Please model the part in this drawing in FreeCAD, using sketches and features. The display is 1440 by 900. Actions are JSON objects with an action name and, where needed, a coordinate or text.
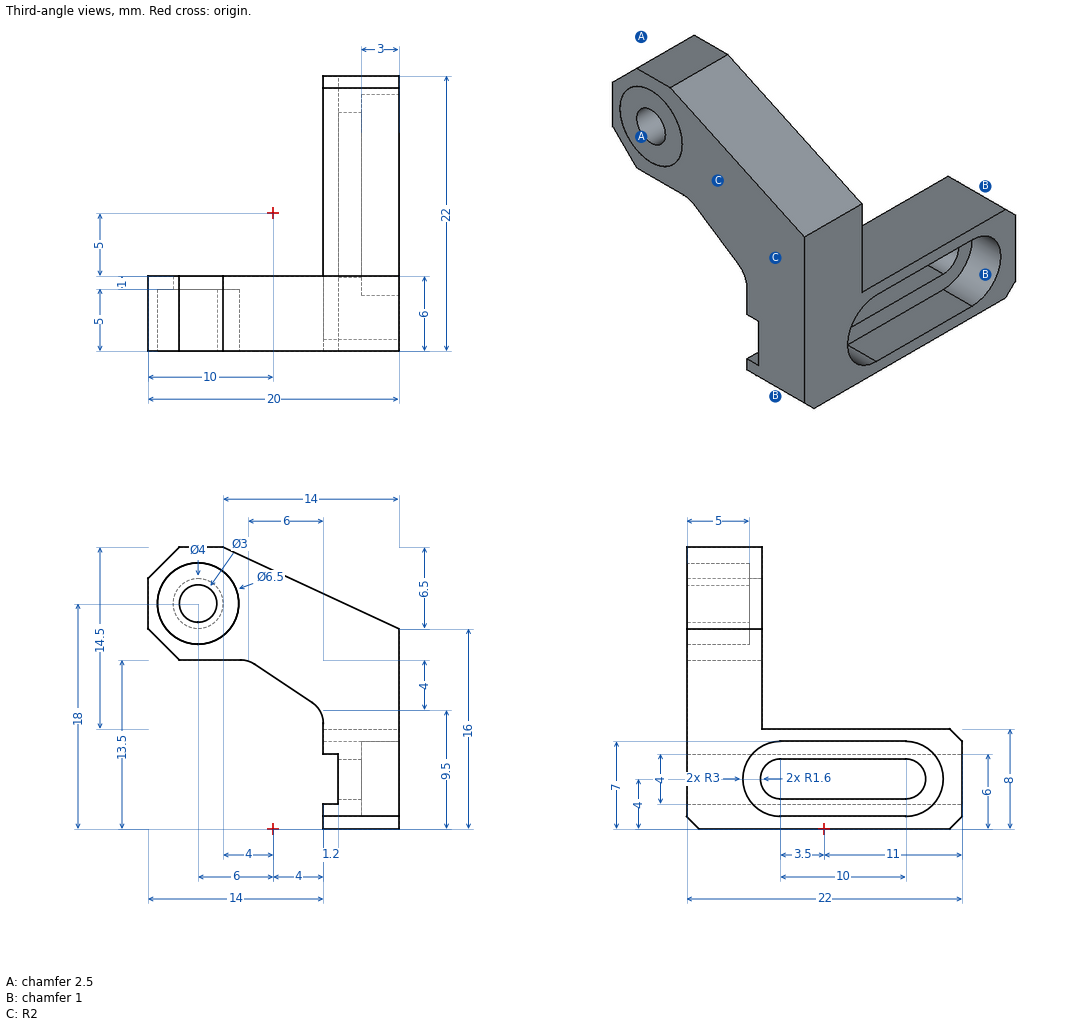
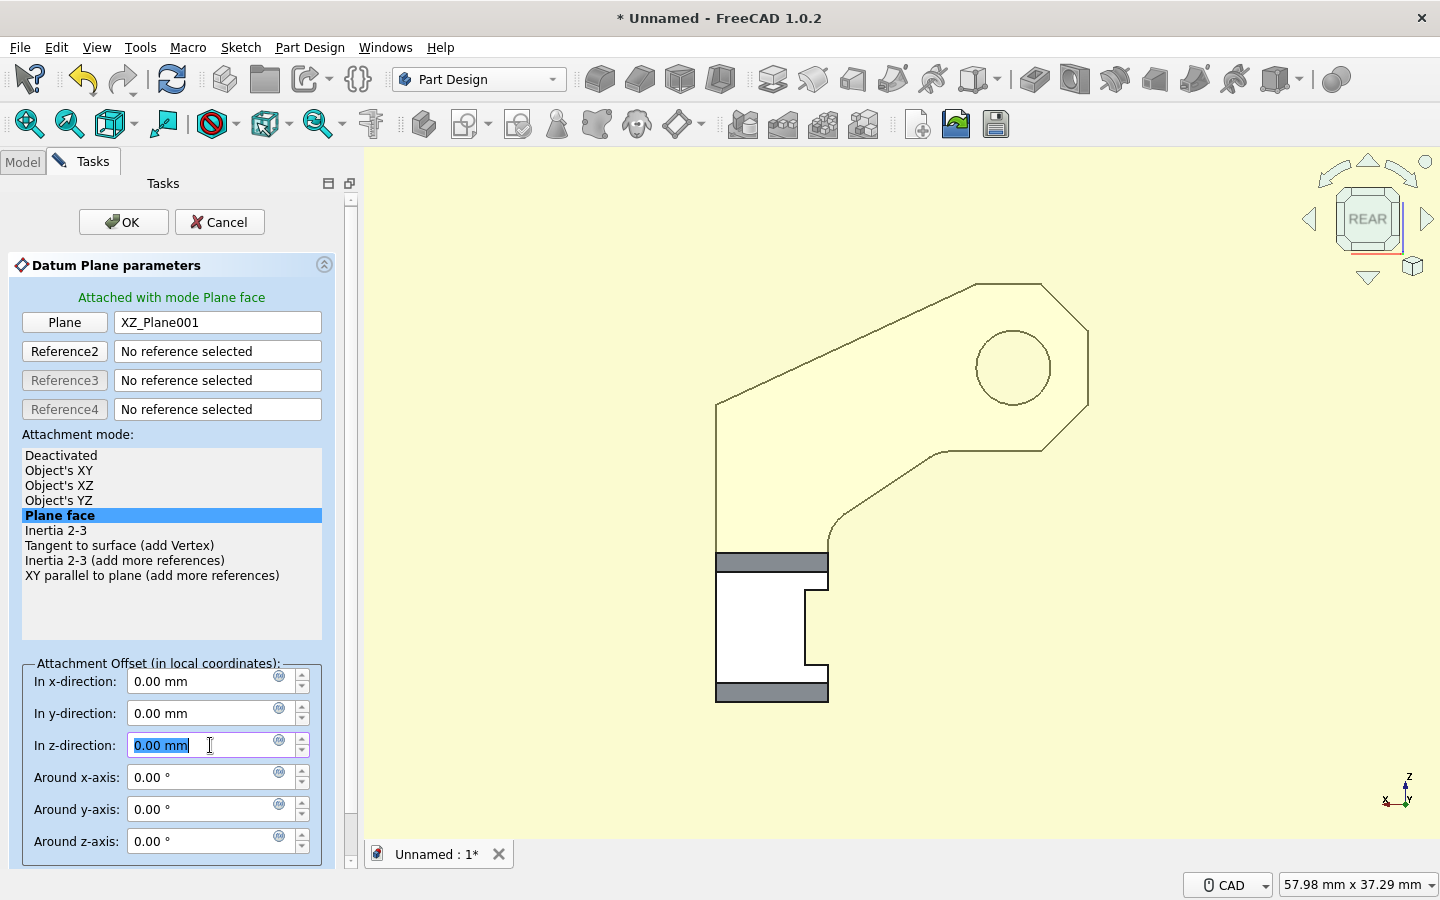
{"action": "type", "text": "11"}
{"action": "key", "text": "Tab"}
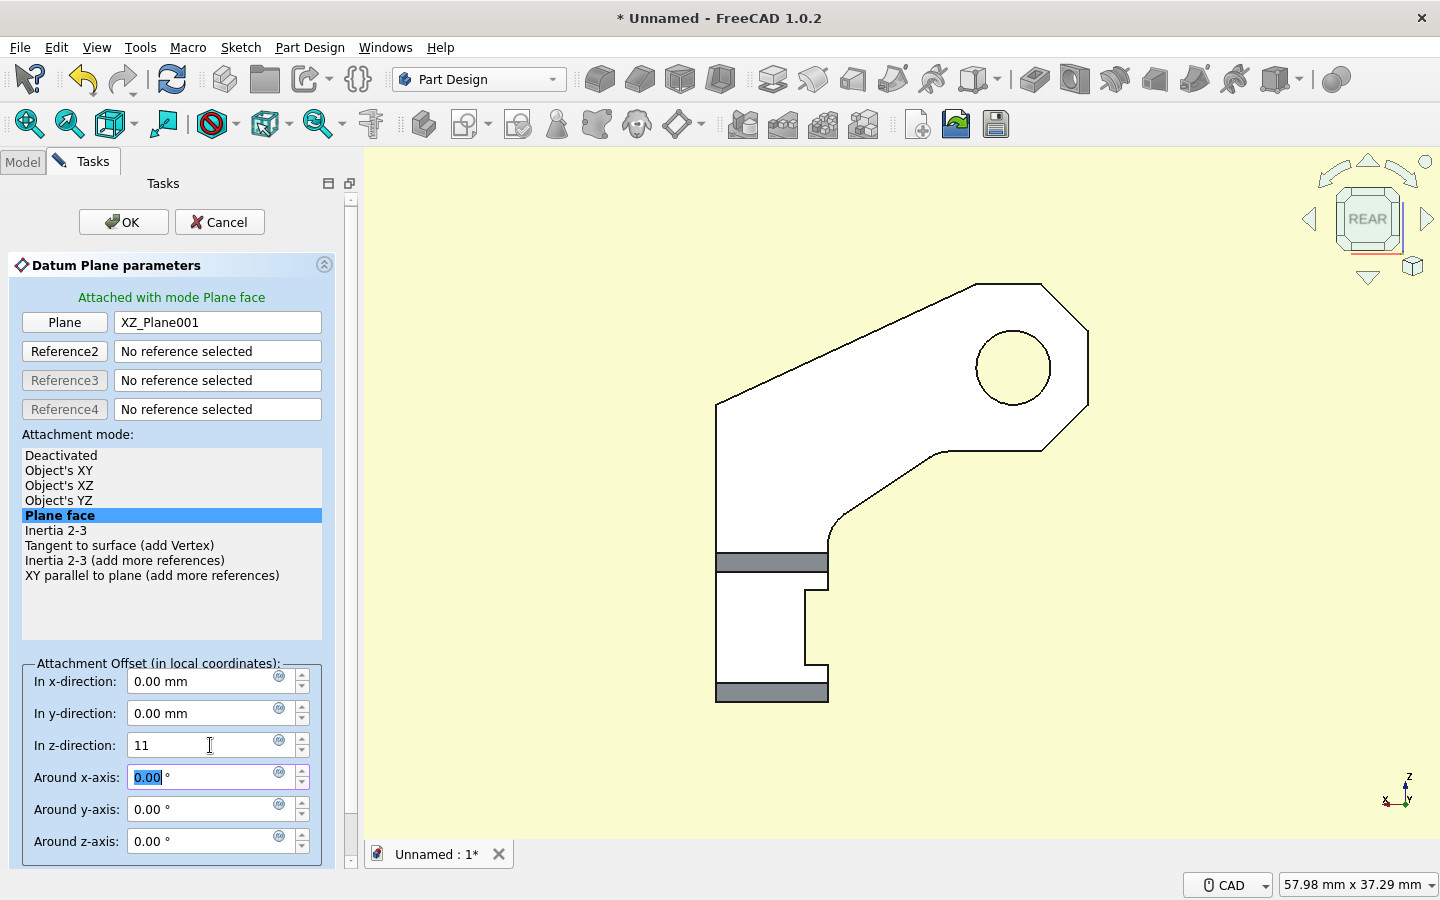
{"action": "left_click", "coordinate": [124, 222]}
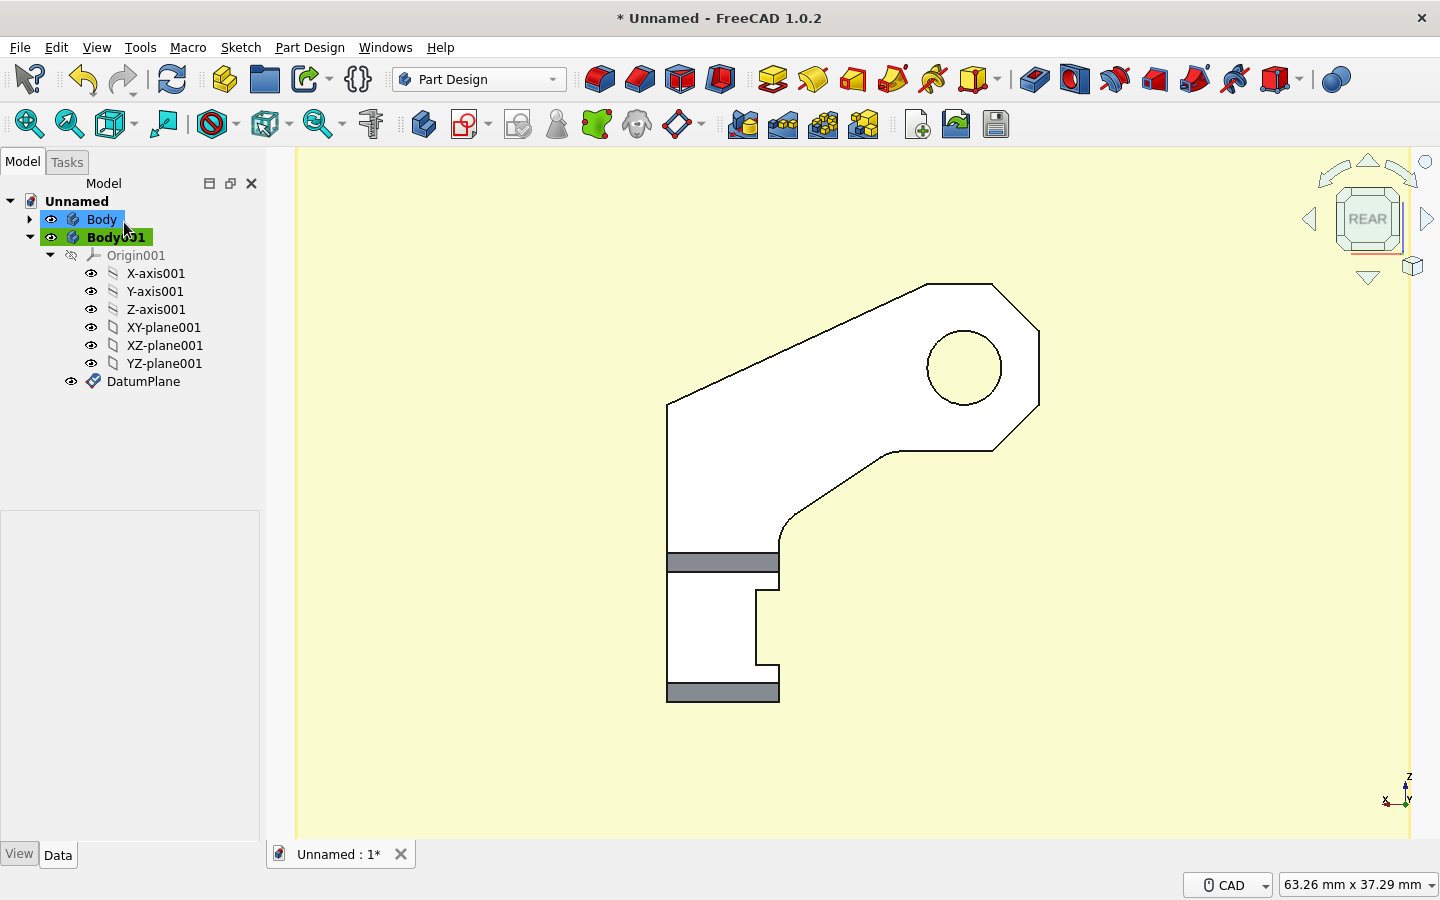
{"action": "left_click", "coordinate": [116, 381]}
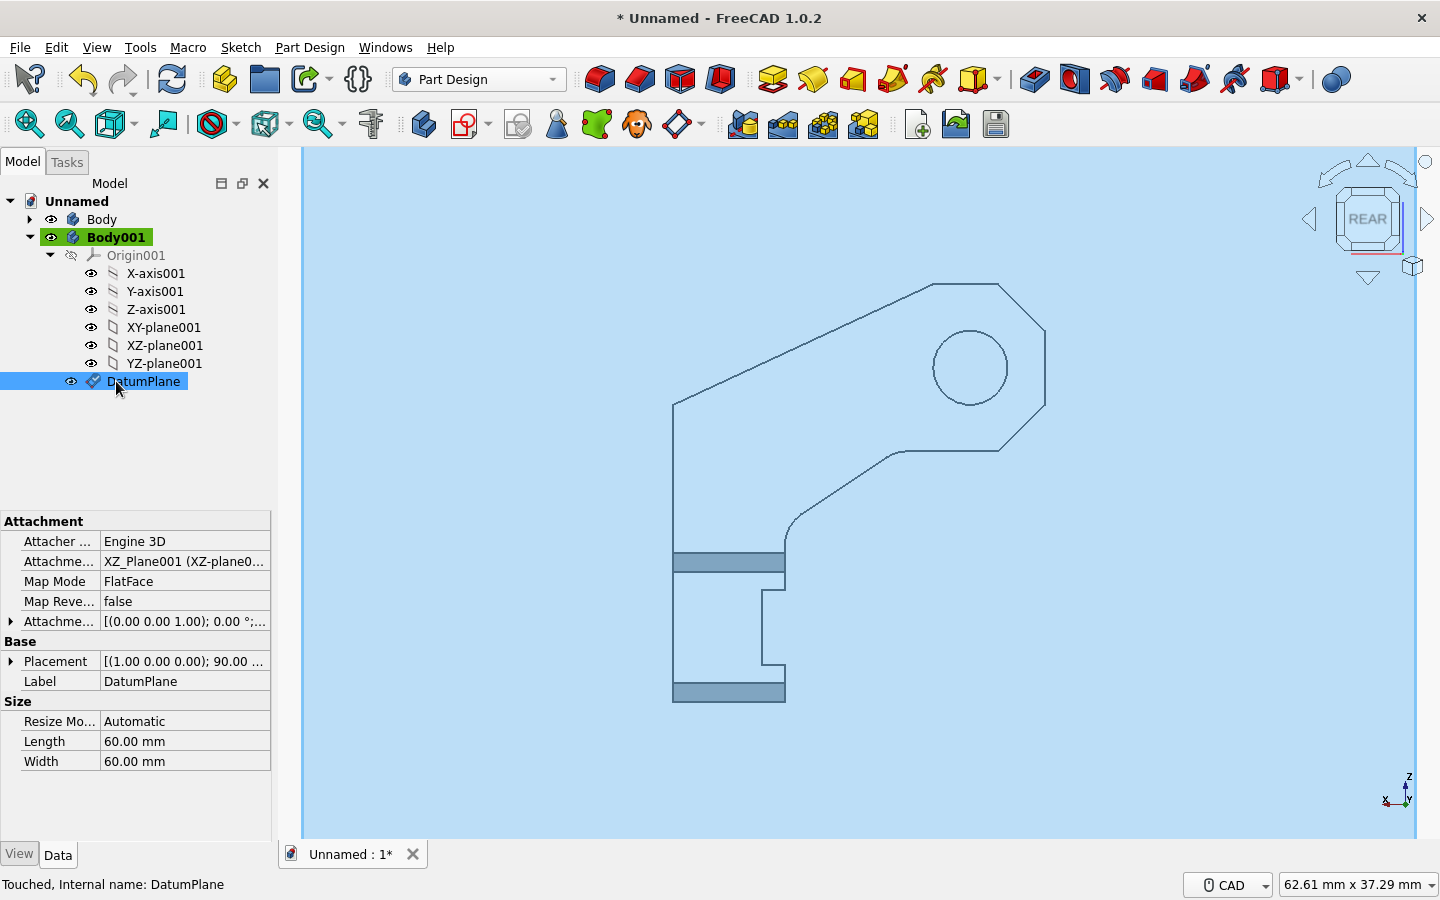
{"action": "left_click", "coordinate": [464, 124]}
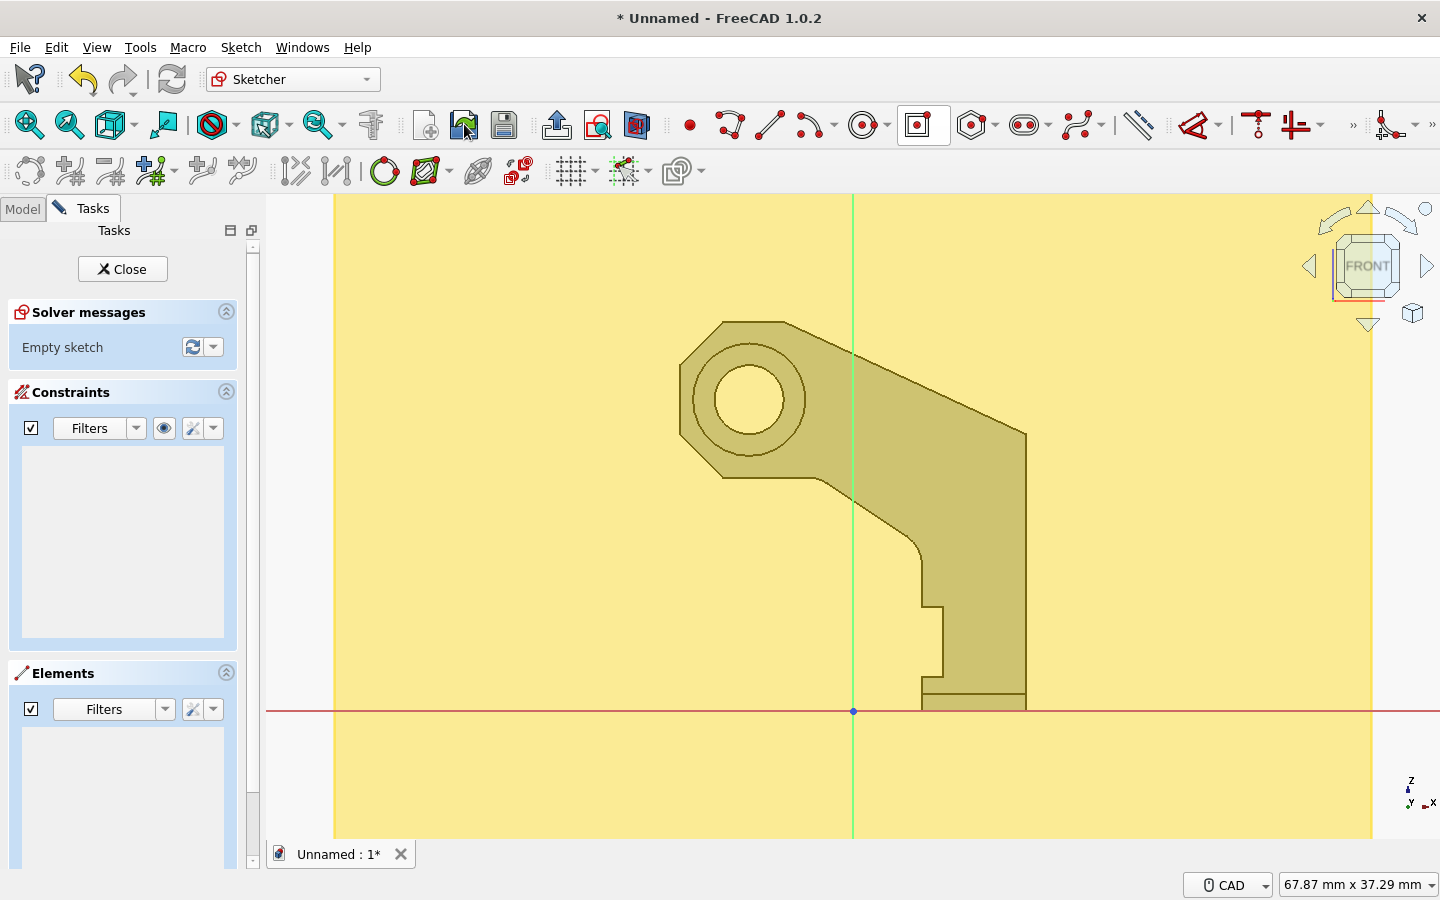
{"action": "scroll", "coordinate": [738, 362], "scroll_direction": "up", "scroll_amount": 7}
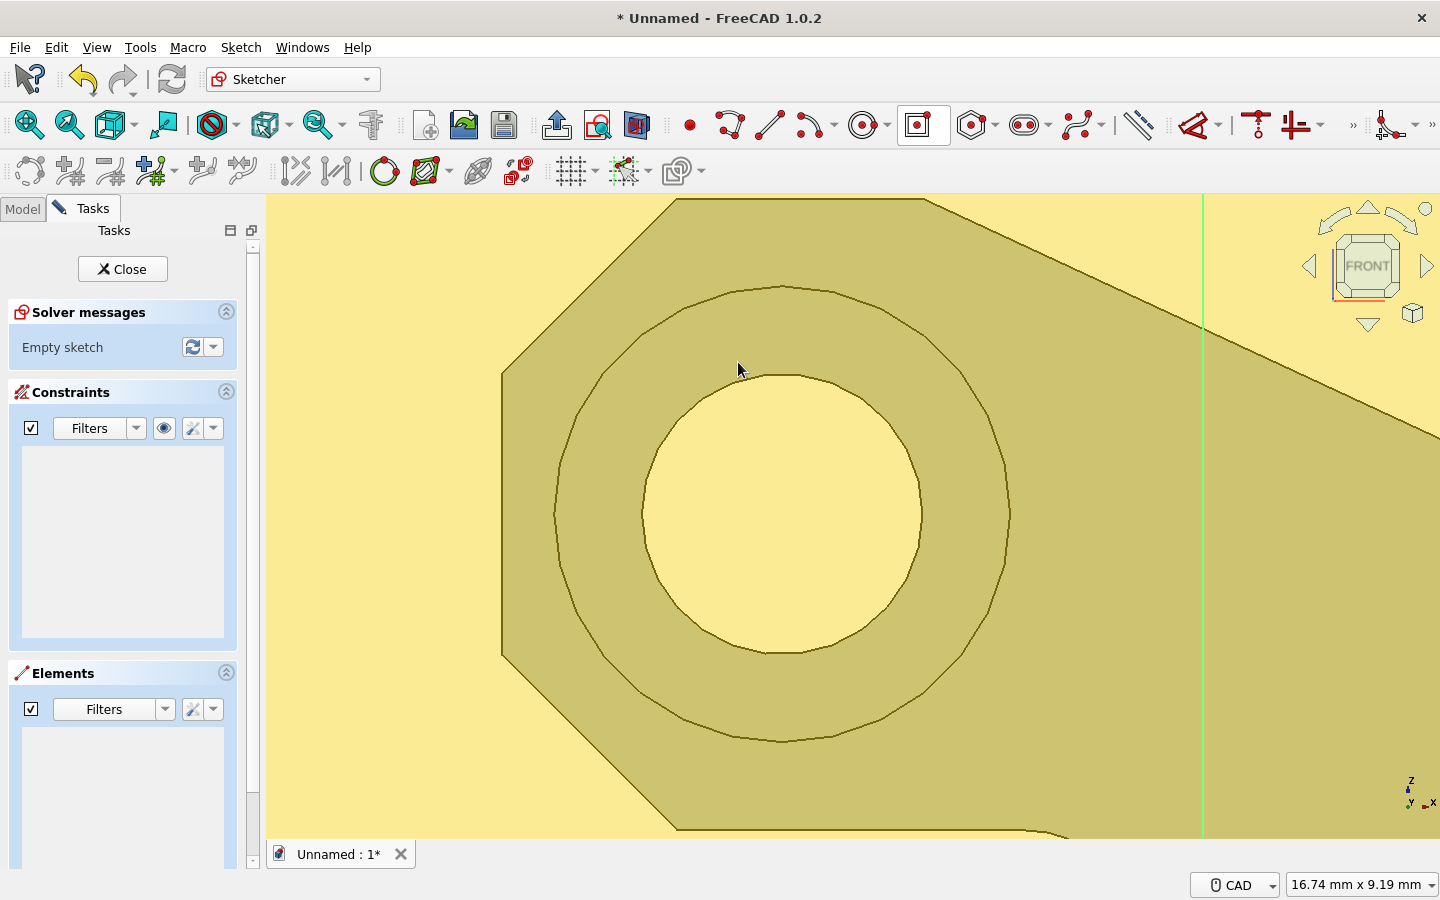
{"action": "left_click", "coordinate": [864, 126]}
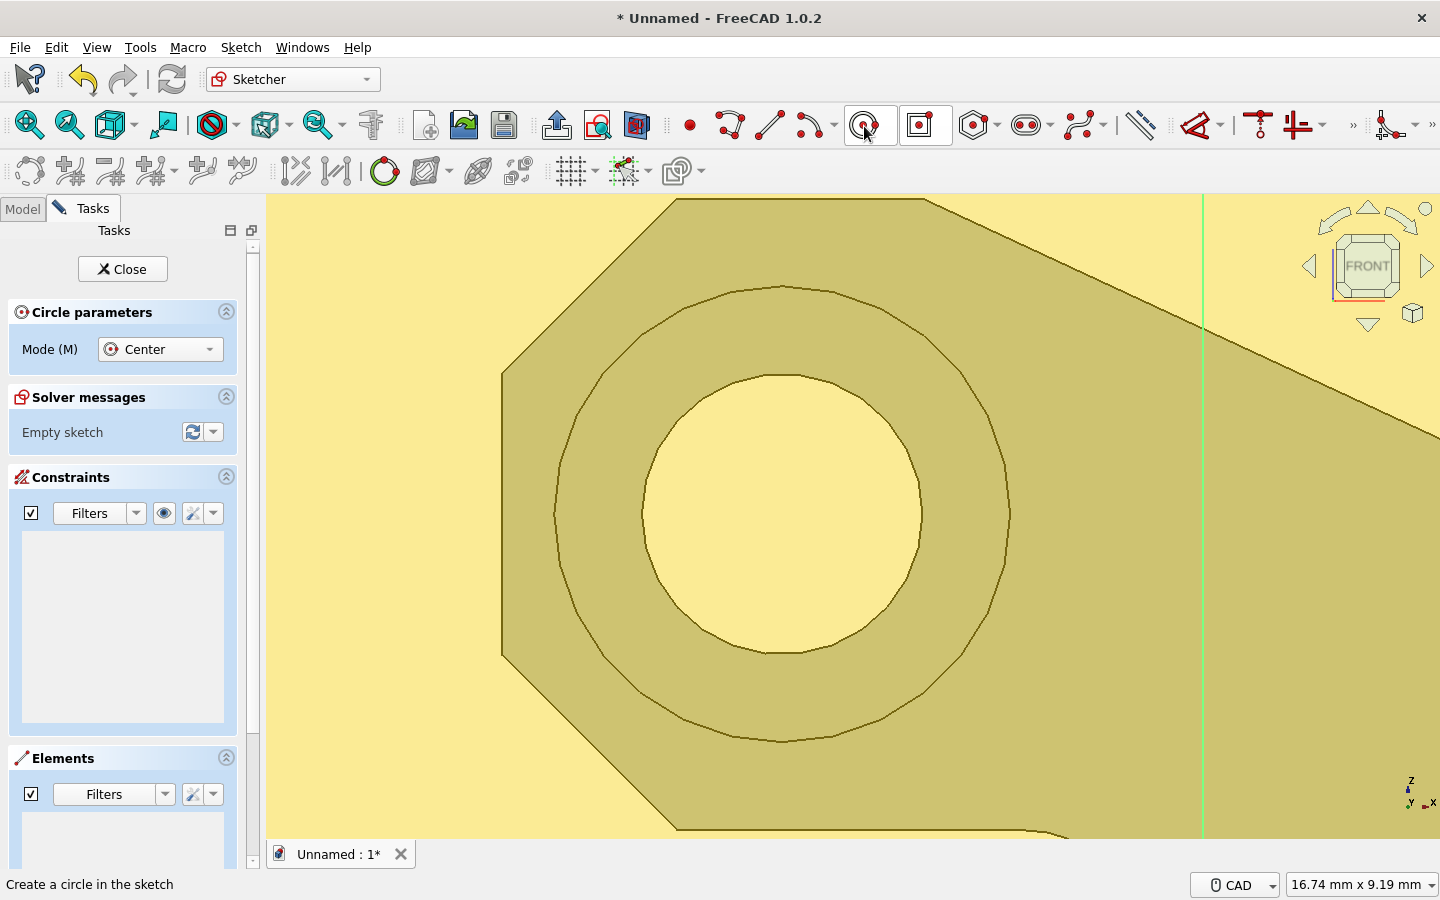
{"action": "left_click", "coordinate": [782, 514]}
{"action": "mouse_move", "coordinate": [943, 353]}